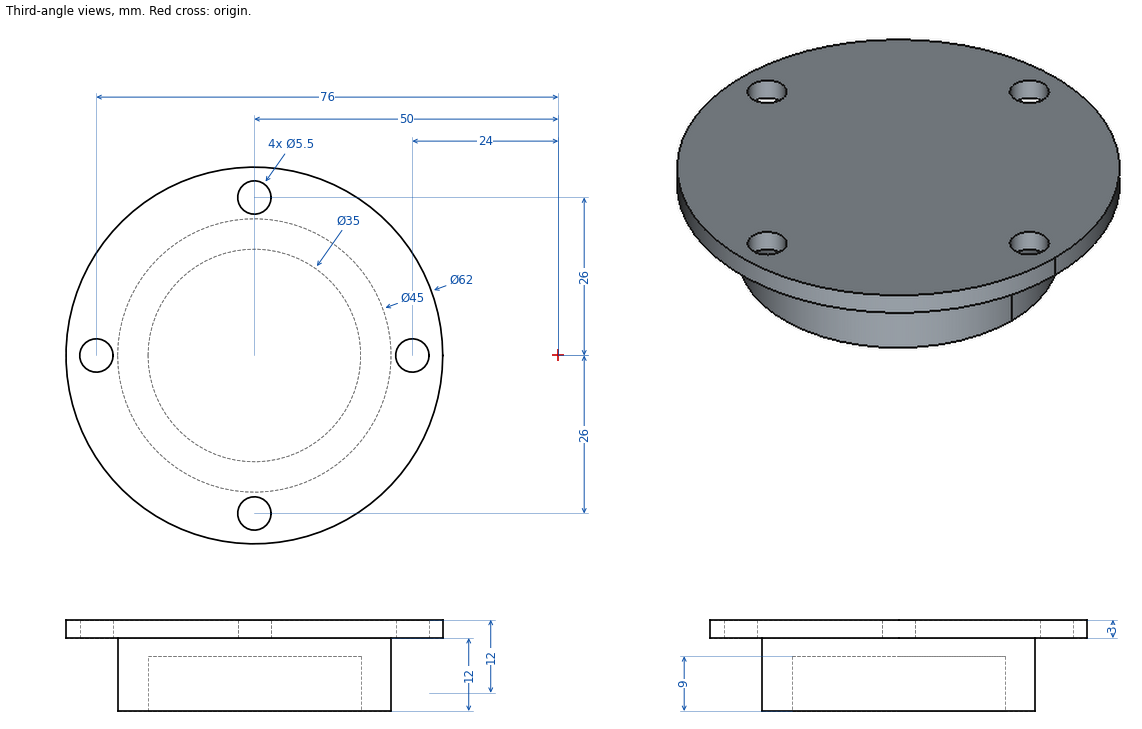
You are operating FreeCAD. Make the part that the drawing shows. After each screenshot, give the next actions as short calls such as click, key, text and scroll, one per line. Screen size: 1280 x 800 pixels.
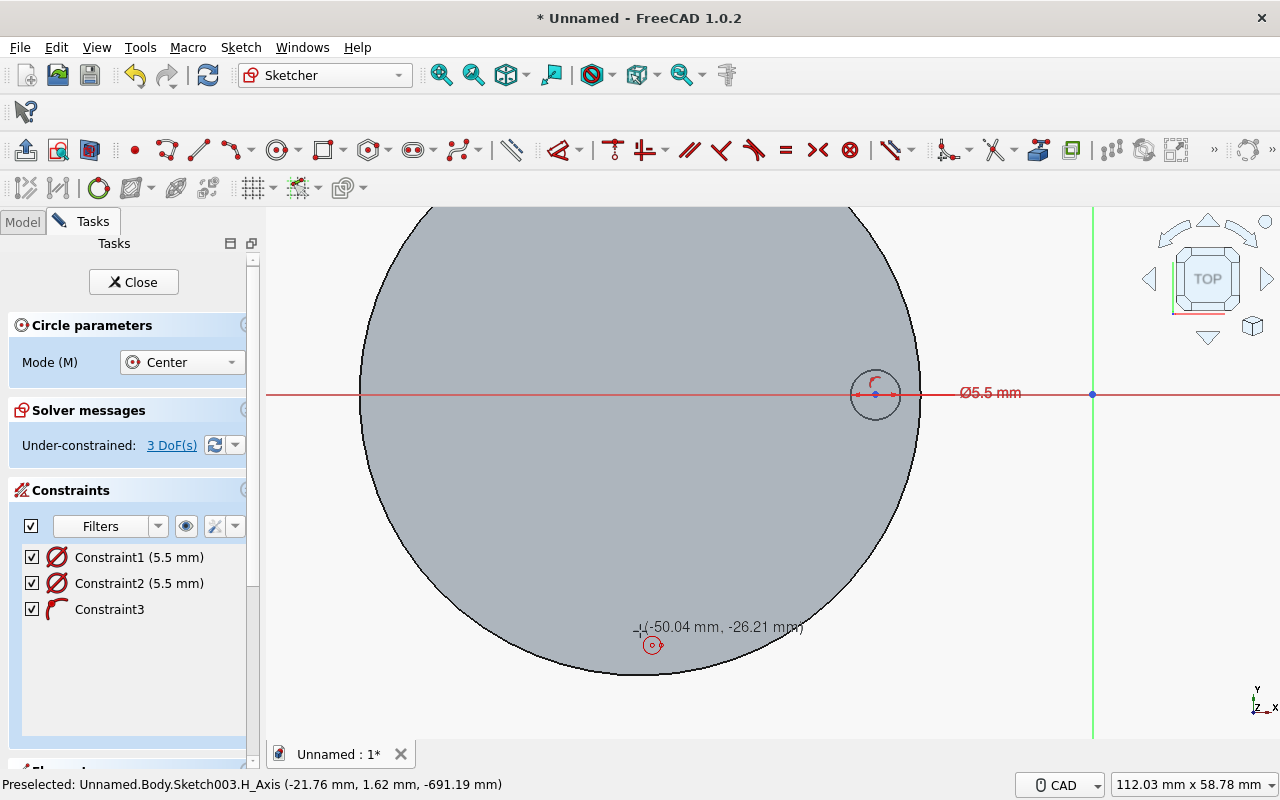
click(640, 630)
move(658, 613)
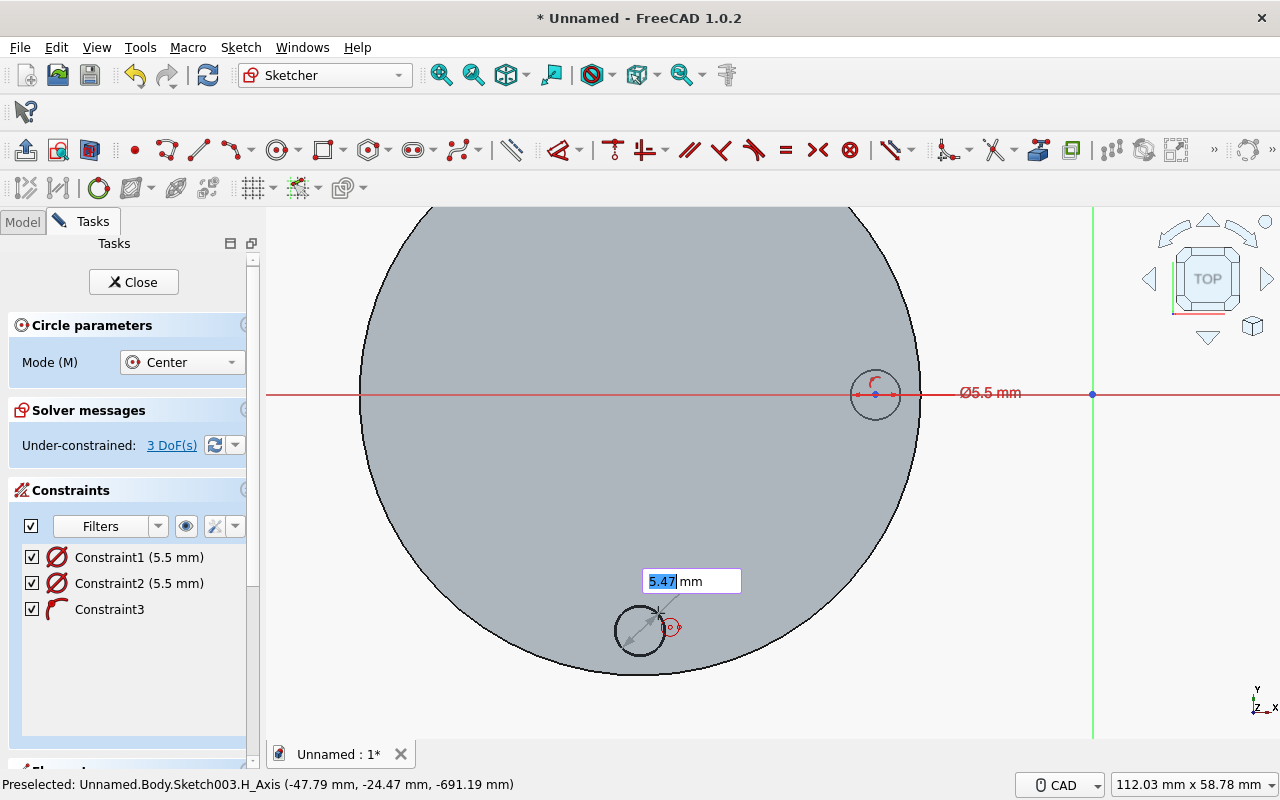
text(5.5)
key(Return)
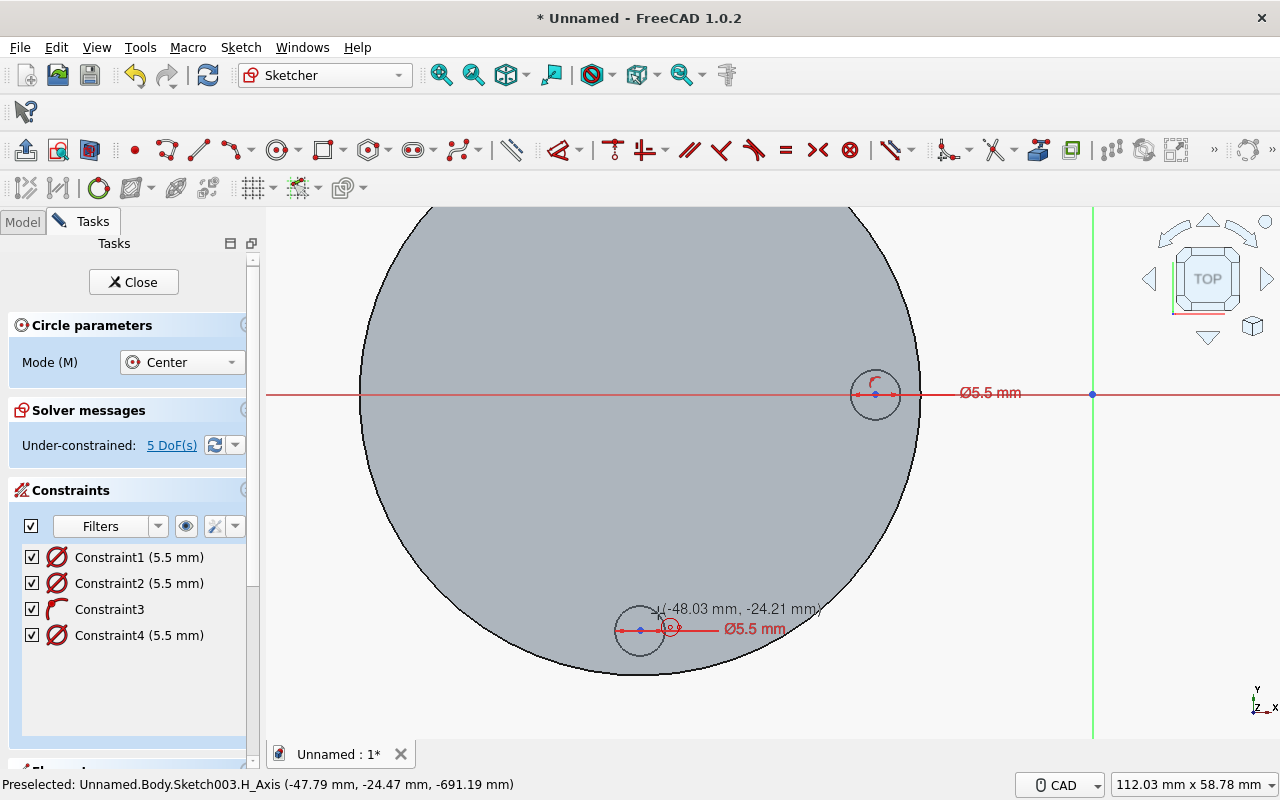
click(405, 395)
move(422, 377)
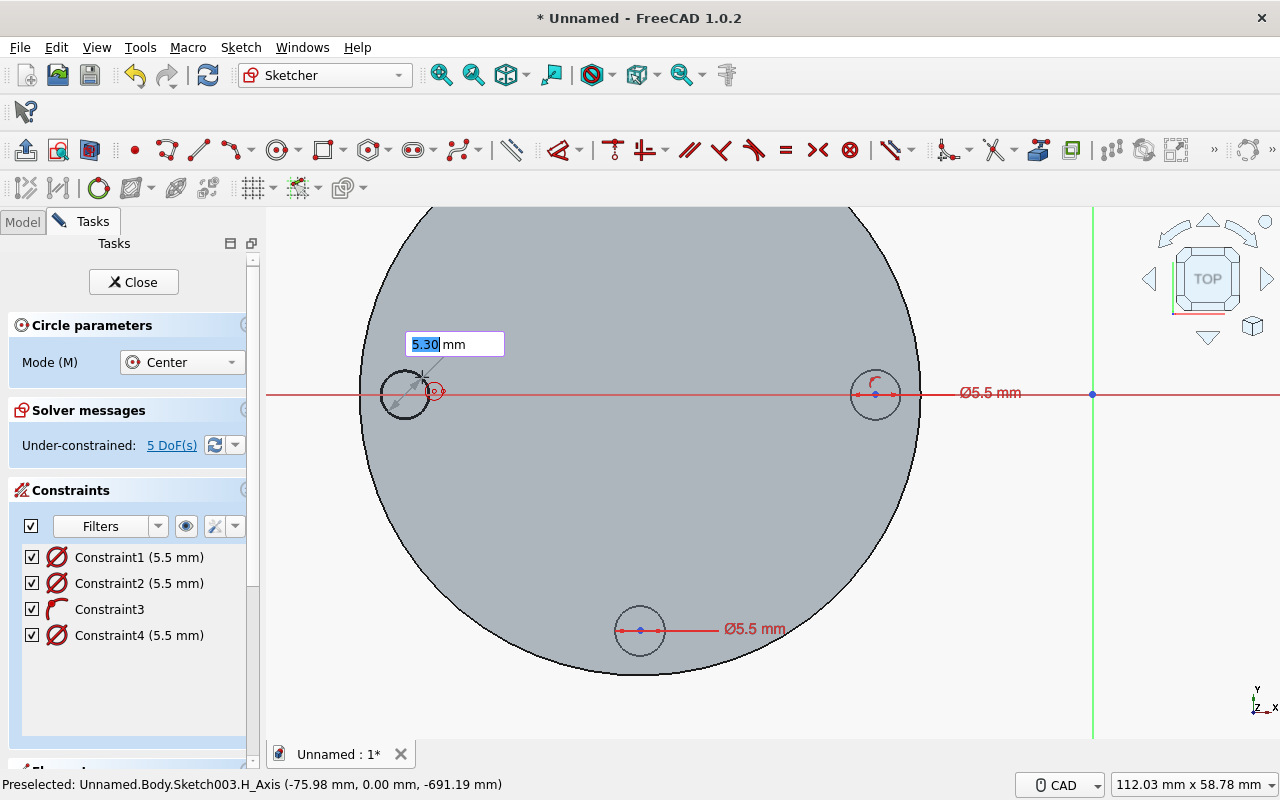
text(5.5)
key(Return)
key(Escape)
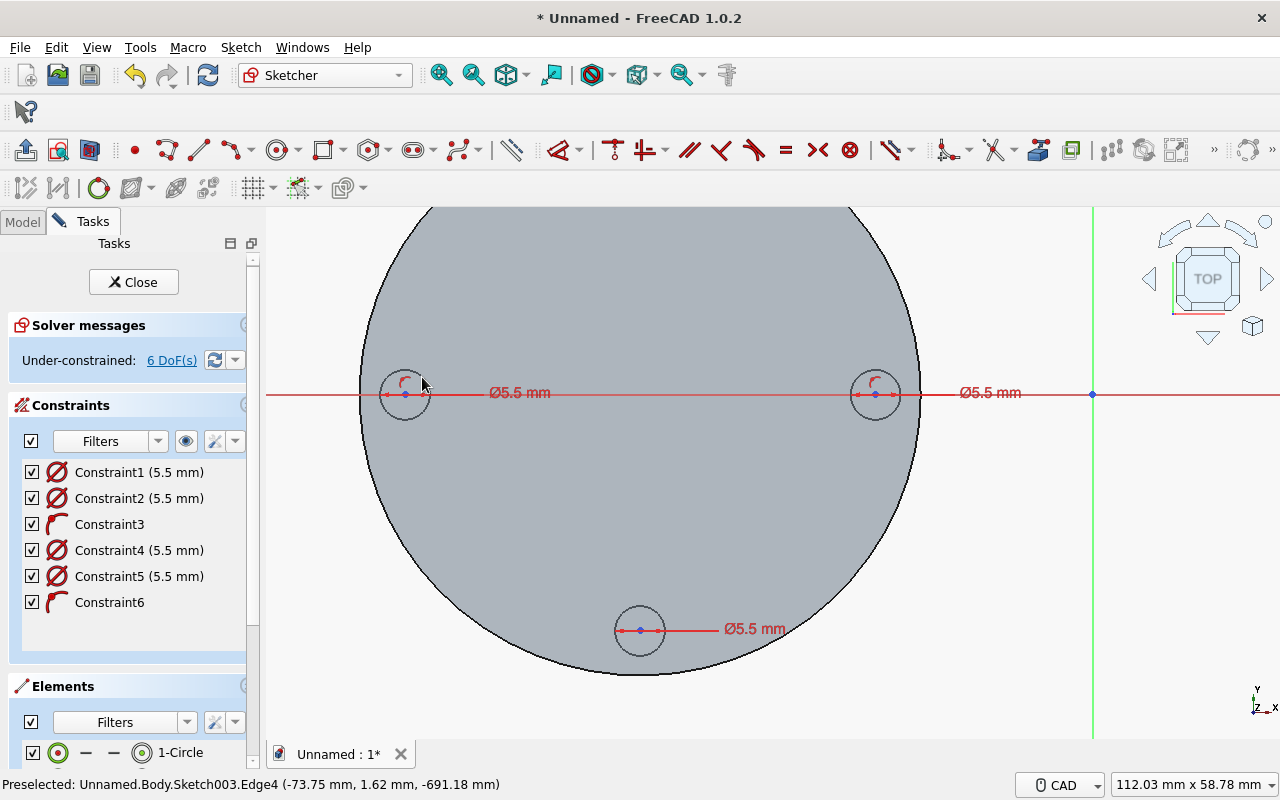
scroll(640, 632, down, 2)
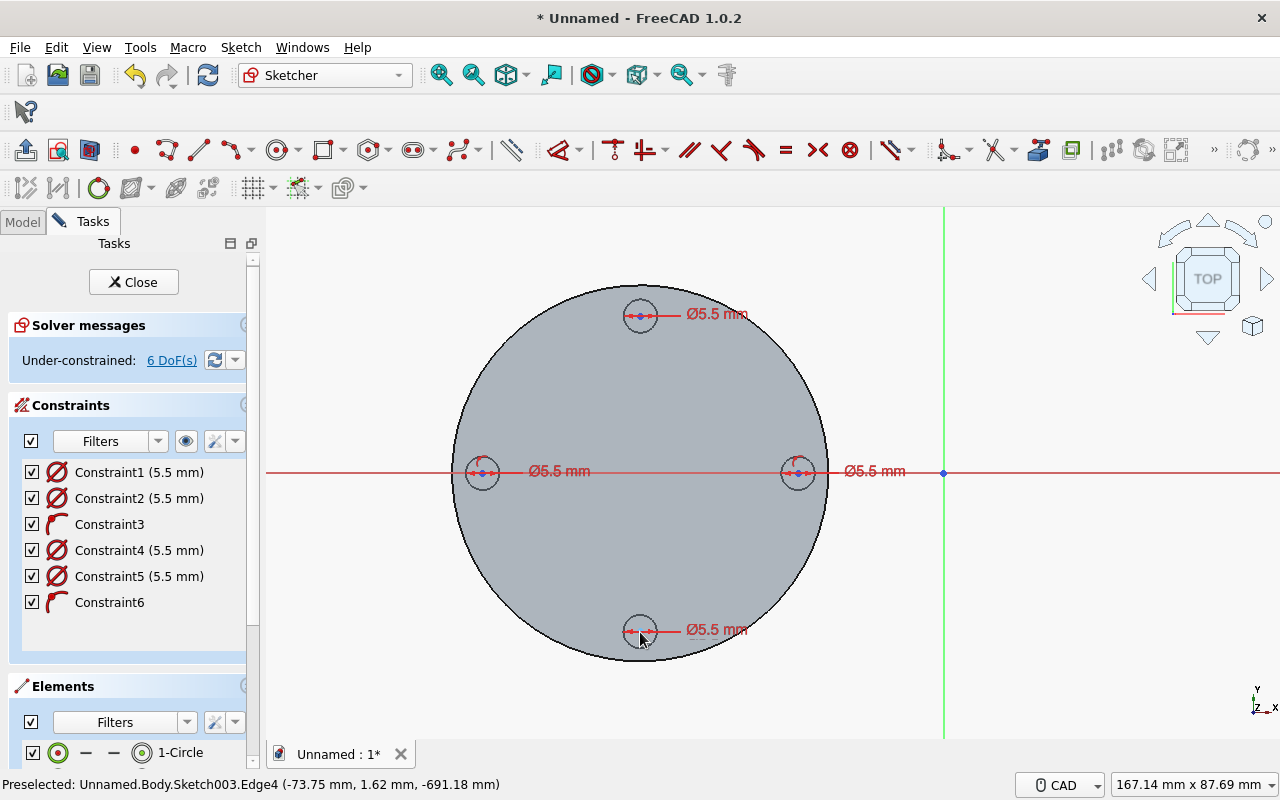
click(641, 316)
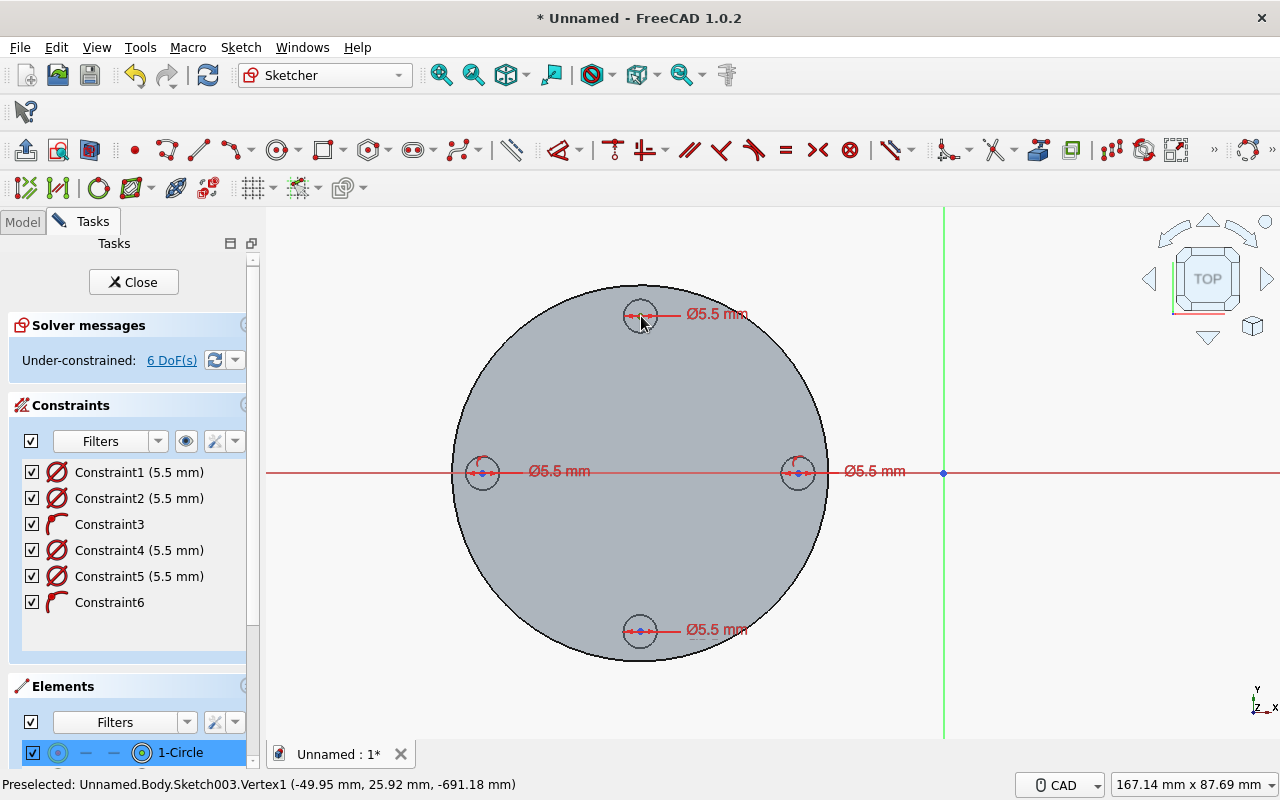
click(640, 632)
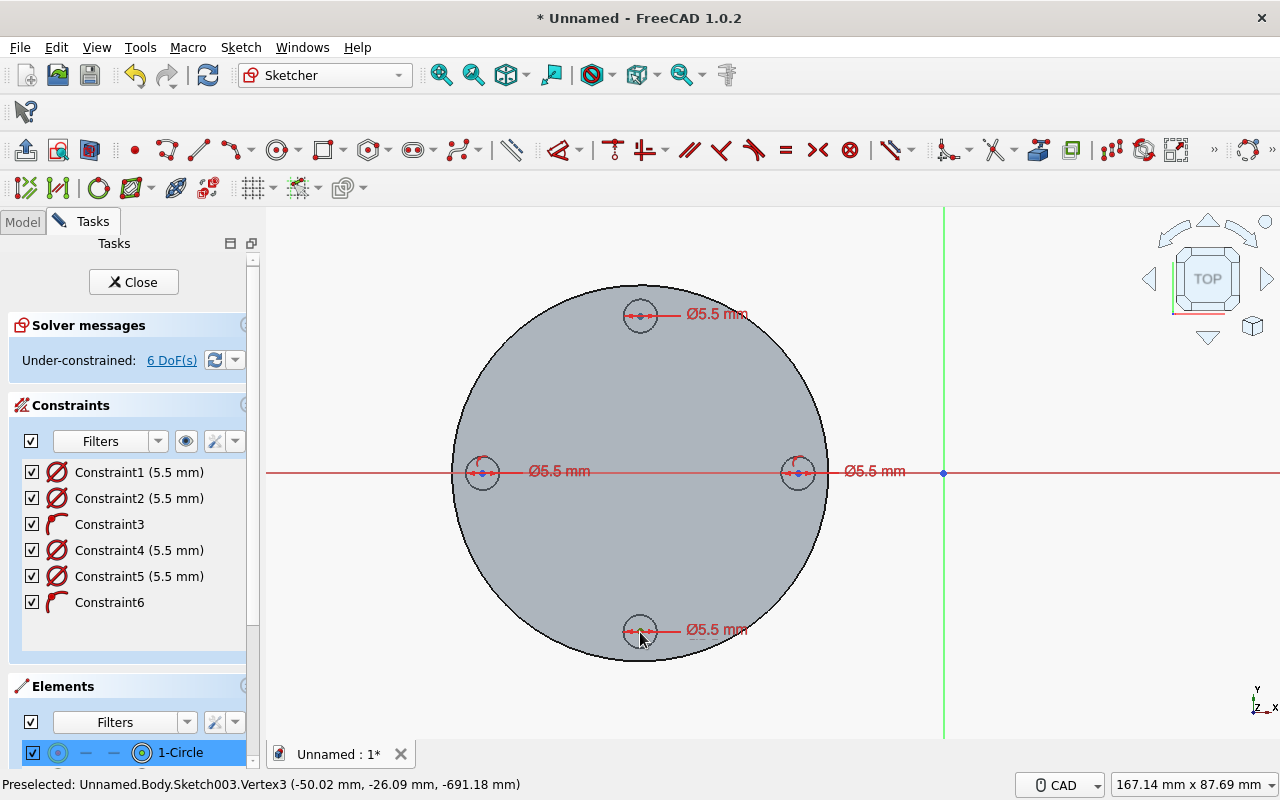
click(668, 150)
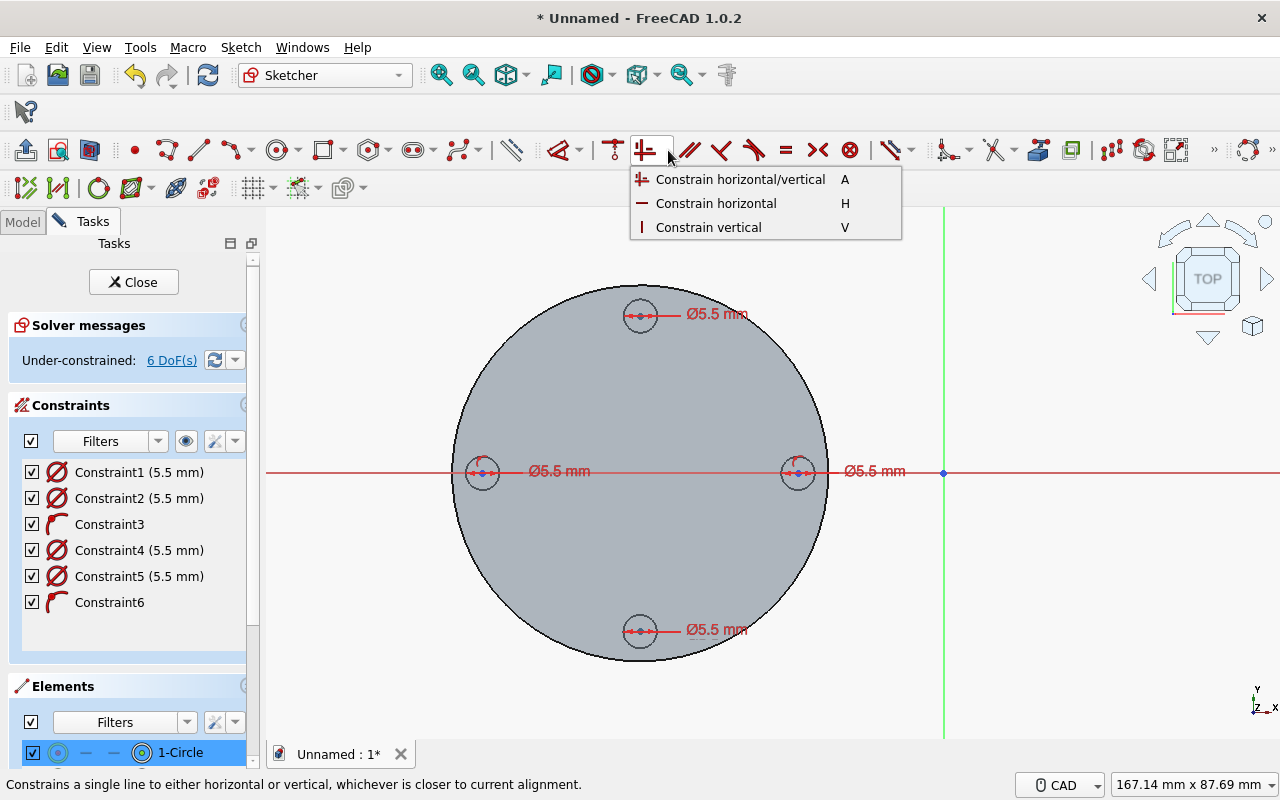
click(766, 227)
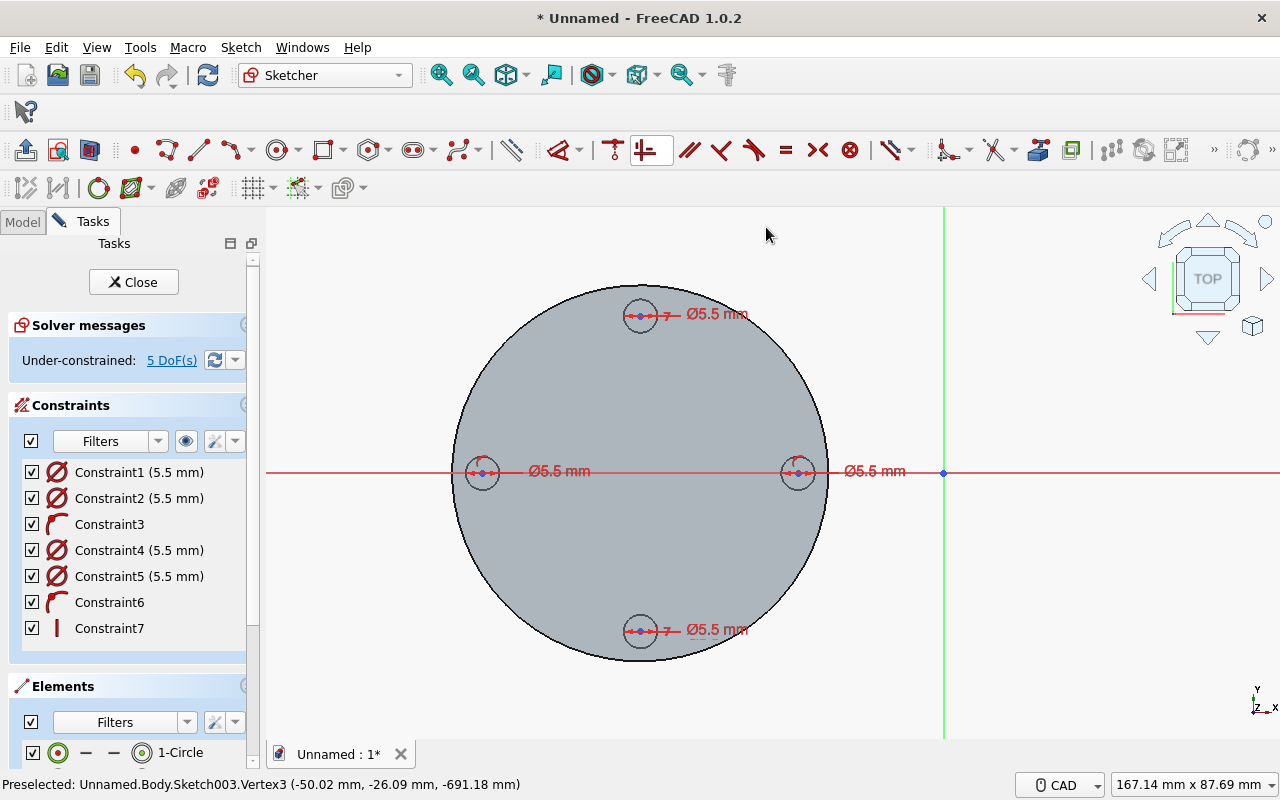
click(558, 150)